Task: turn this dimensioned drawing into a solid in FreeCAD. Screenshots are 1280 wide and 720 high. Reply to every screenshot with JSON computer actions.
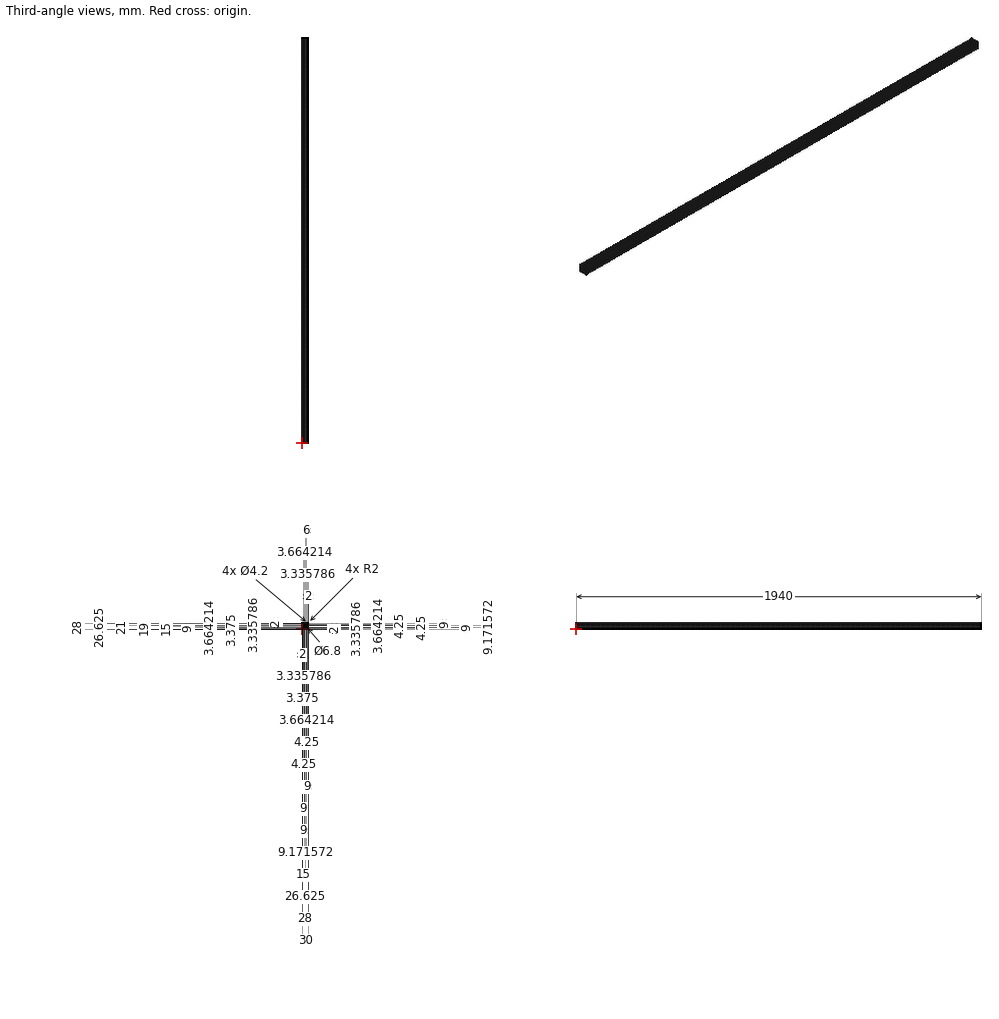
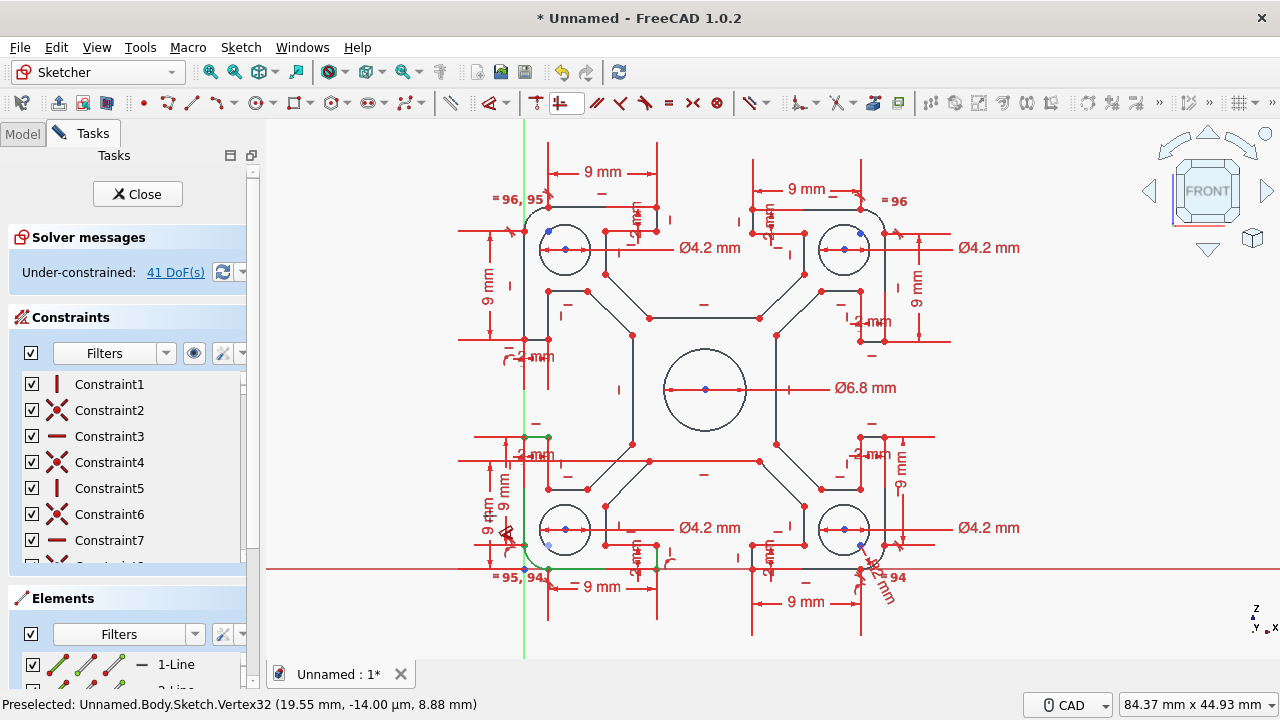
{"action": "left_click", "coordinate": [633, 445]}
{"action": "left_click", "coordinate": [579, 411]}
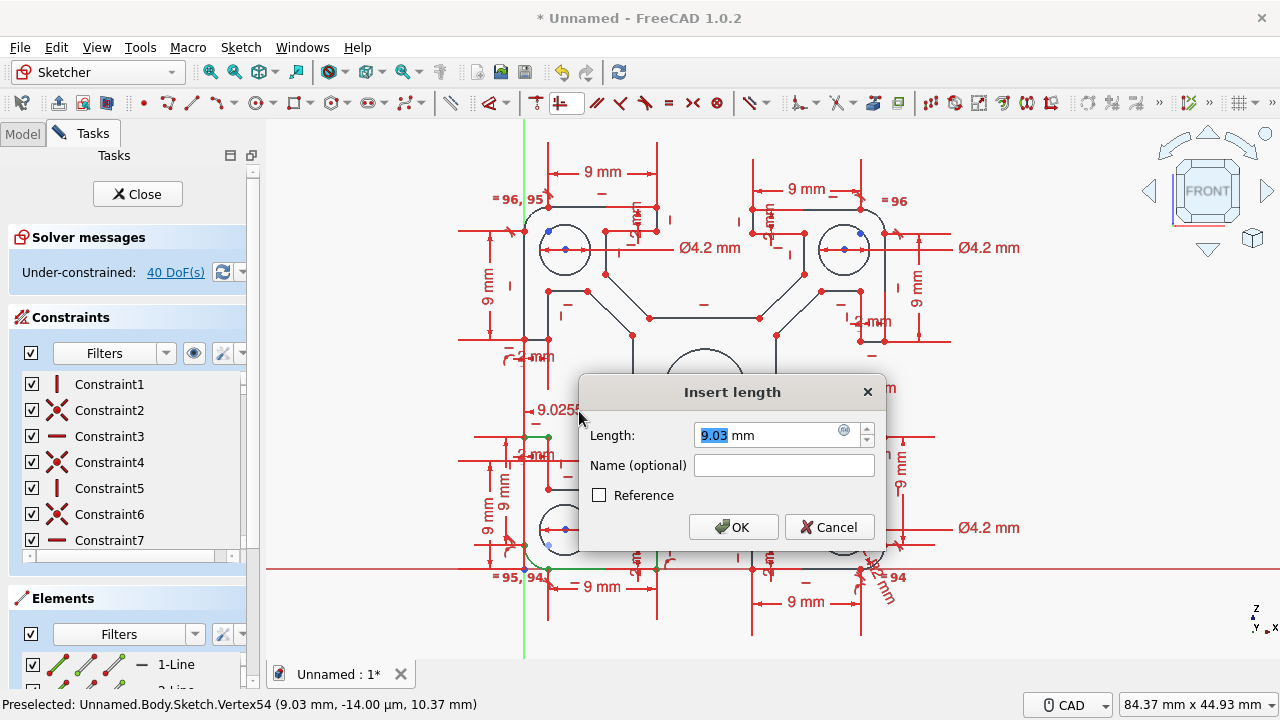
{"action": "type", "text": "9"}
{"action": "key", "text": "Return"}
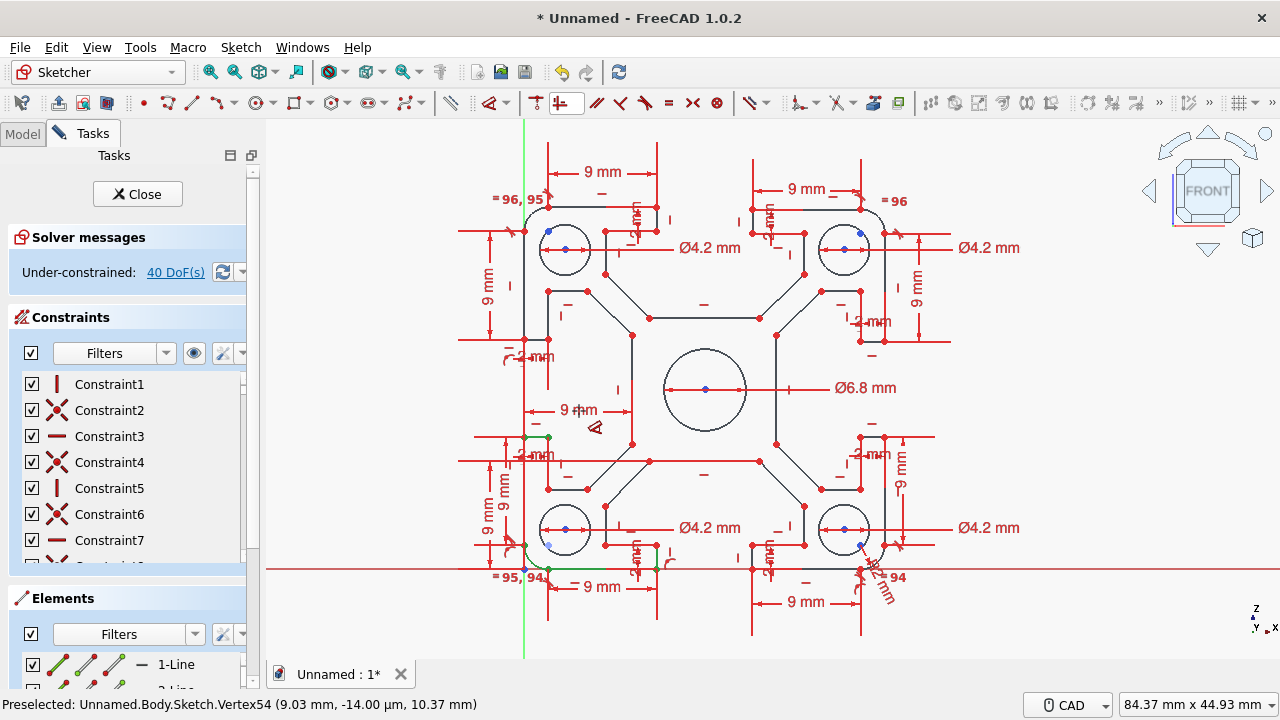
{"action": "left_click", "coordinate": [705, 390]}
{"action": "left_click", "coordinate": [678, 603]}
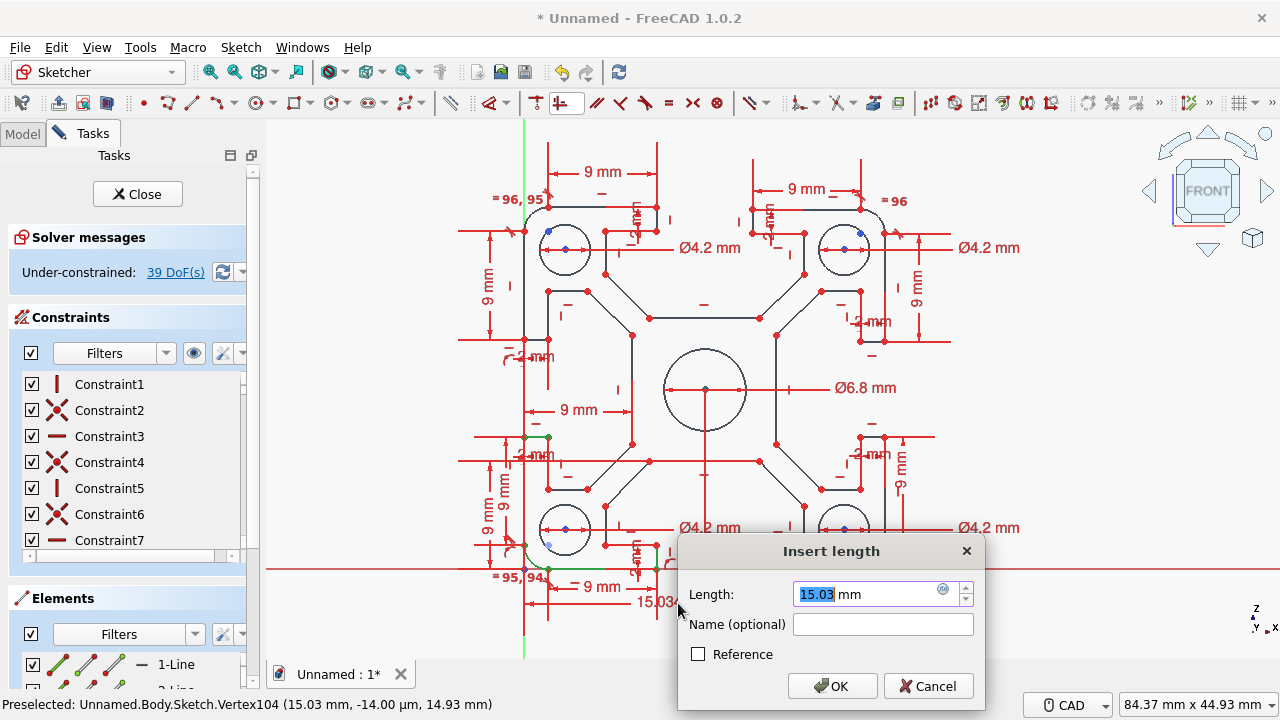
{"action": "type", "text": "15"}
{"action": "key", "text": "Return"}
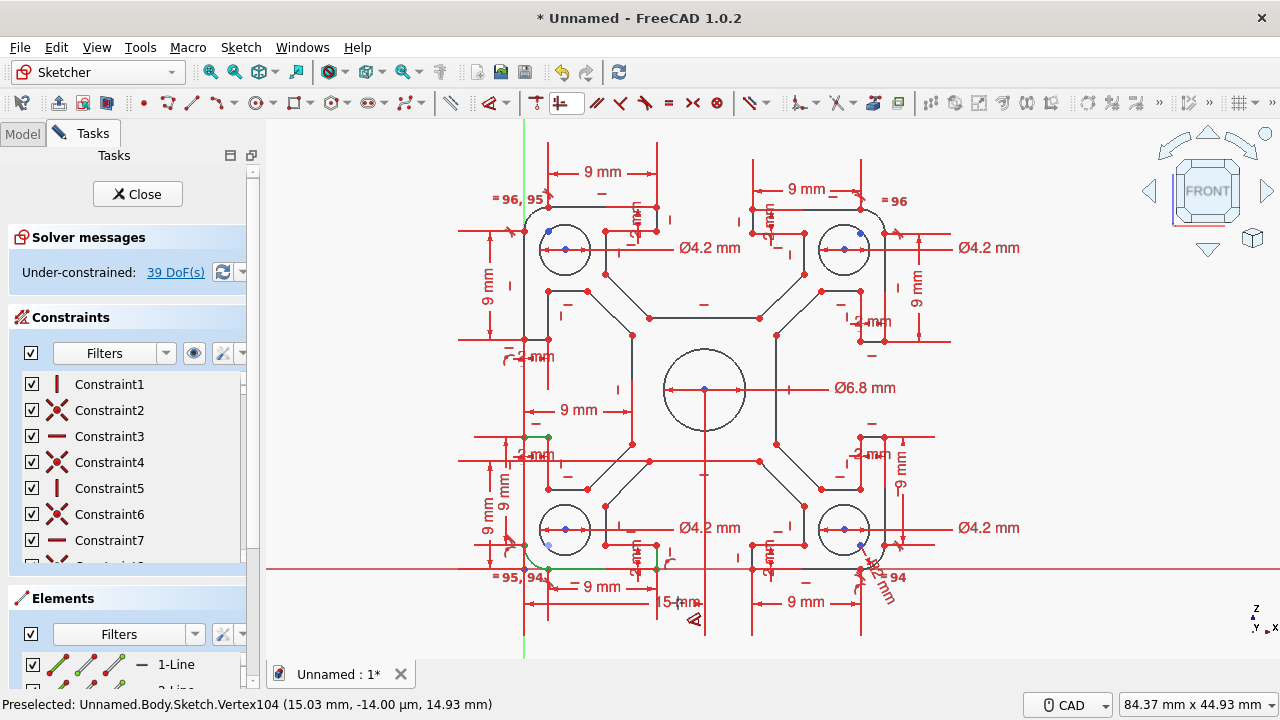
{"action": "left_click", "coordinate": [705, 390]}
{"action": "left_click", "coordinate": [490, 417]}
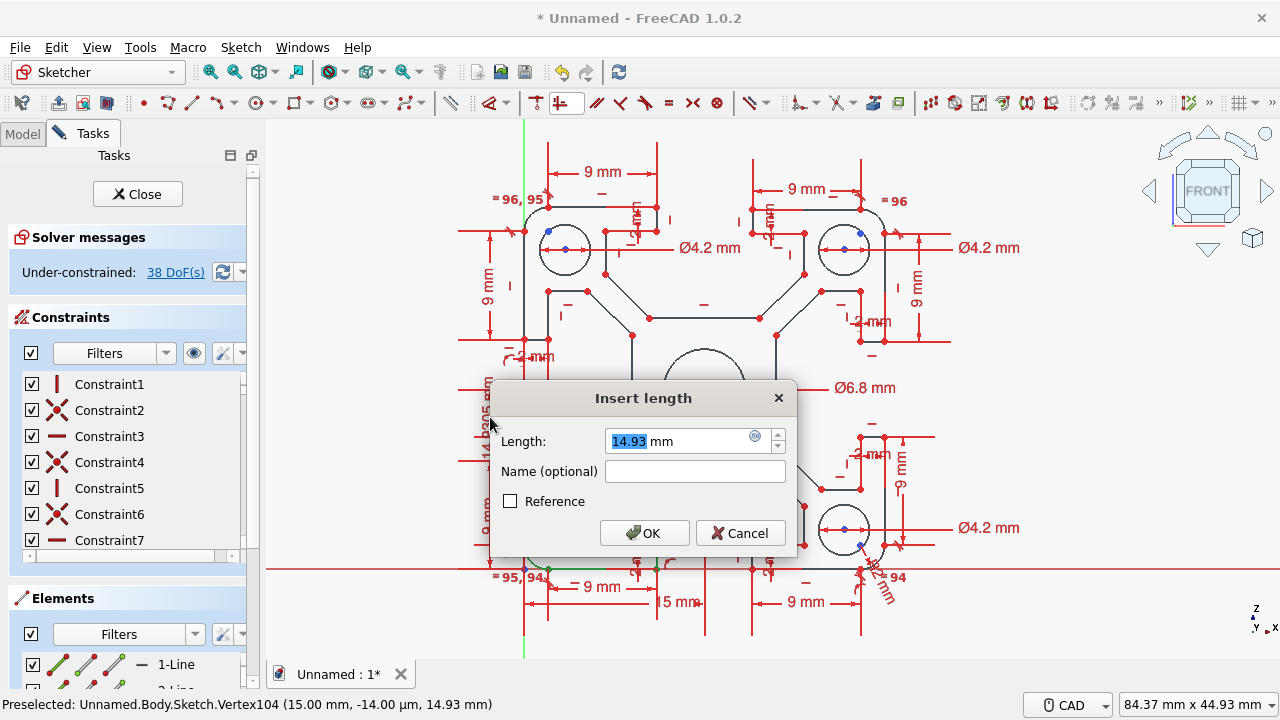
{"action": "type", "text": "15"}
{"action": "key", "text": "Return"}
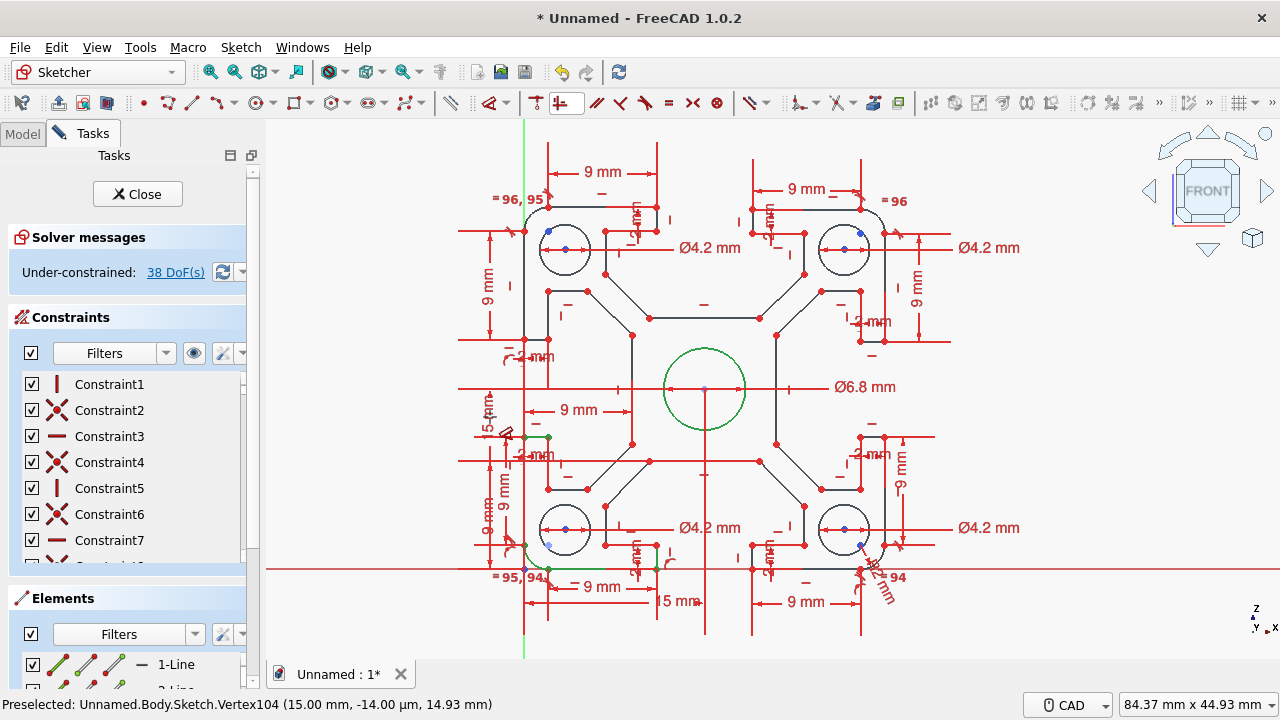
{"action": "left_click", "coordinate": [776, 335]}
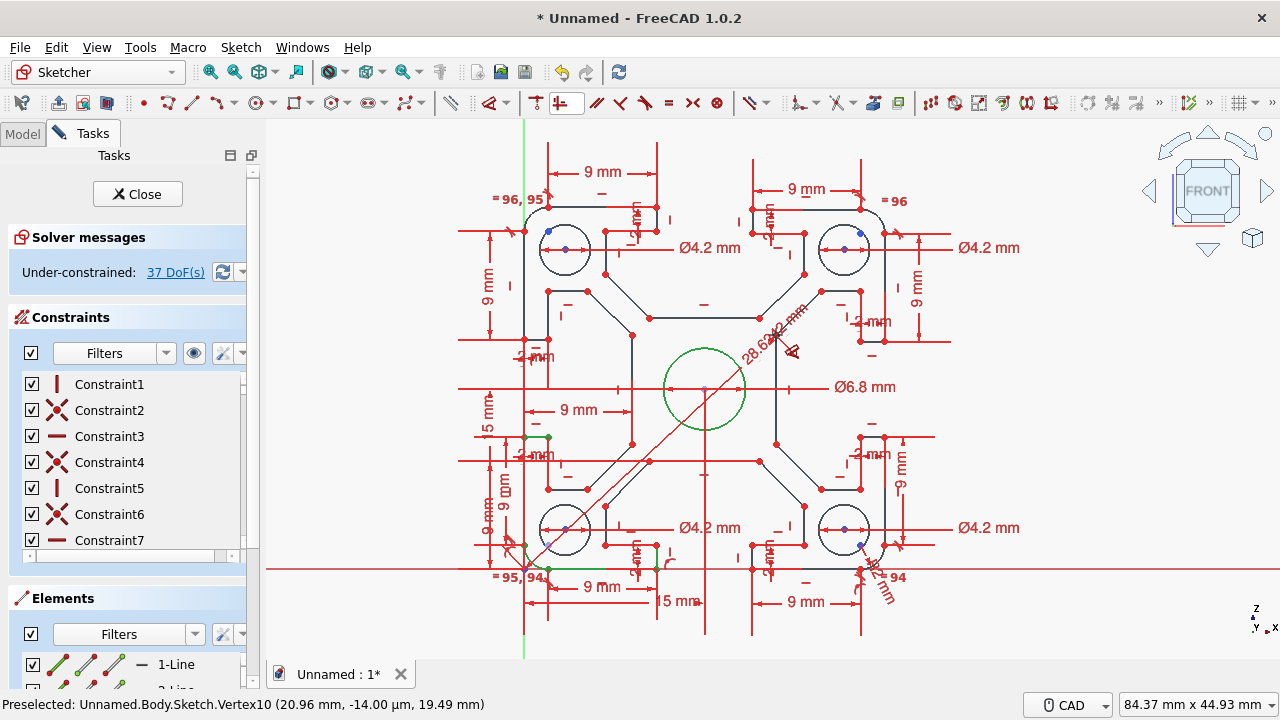
{"action": "left_click", "coordinate": [705, 389]}
{"action": "left_click", "coordinate": [740, 301]}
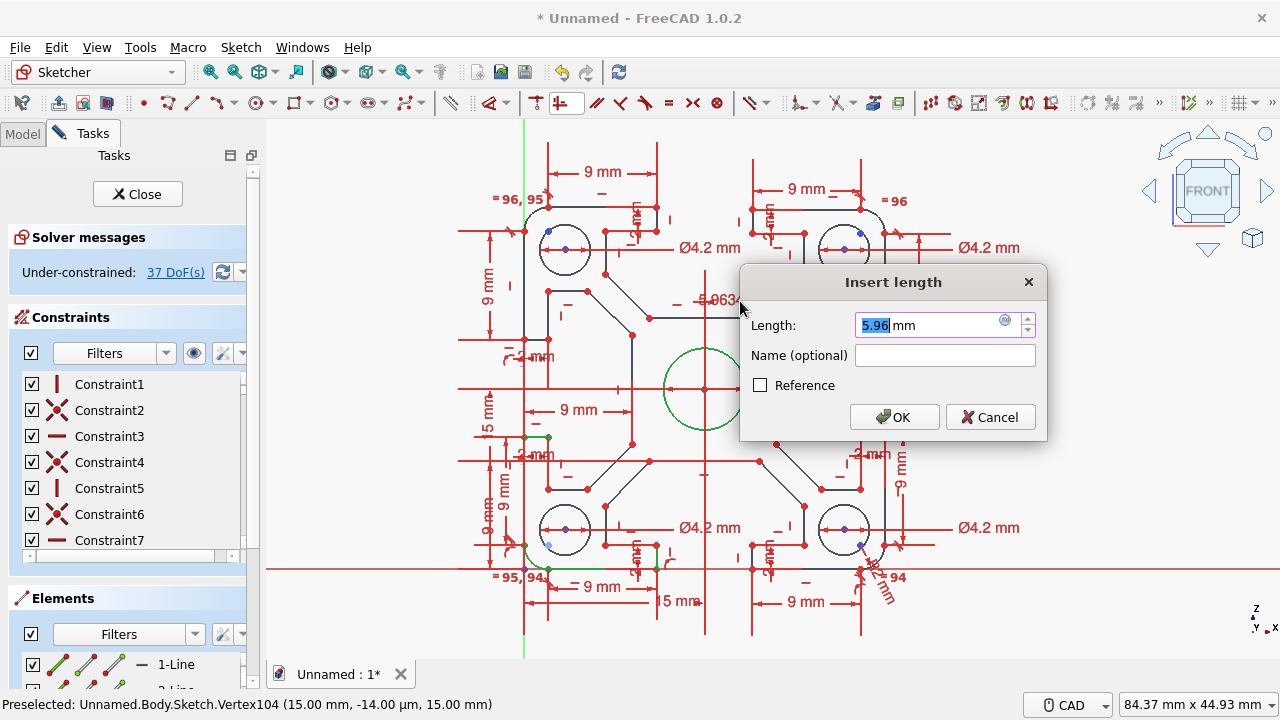
{"action": "type", "text": "6"}
{"action": "key", "text": "Return"}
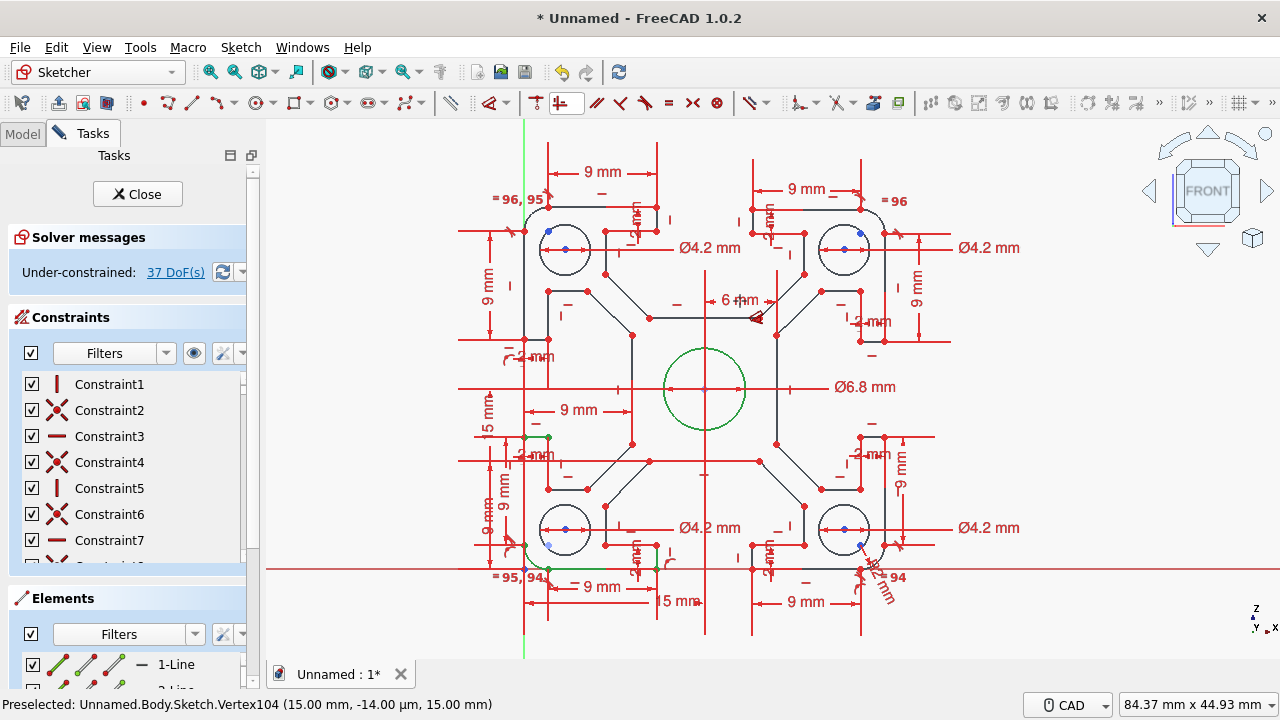
{"action": "left_click", "coordinate": [885, 234]}
{"action": "left_click", "coordinate": [705, 200]}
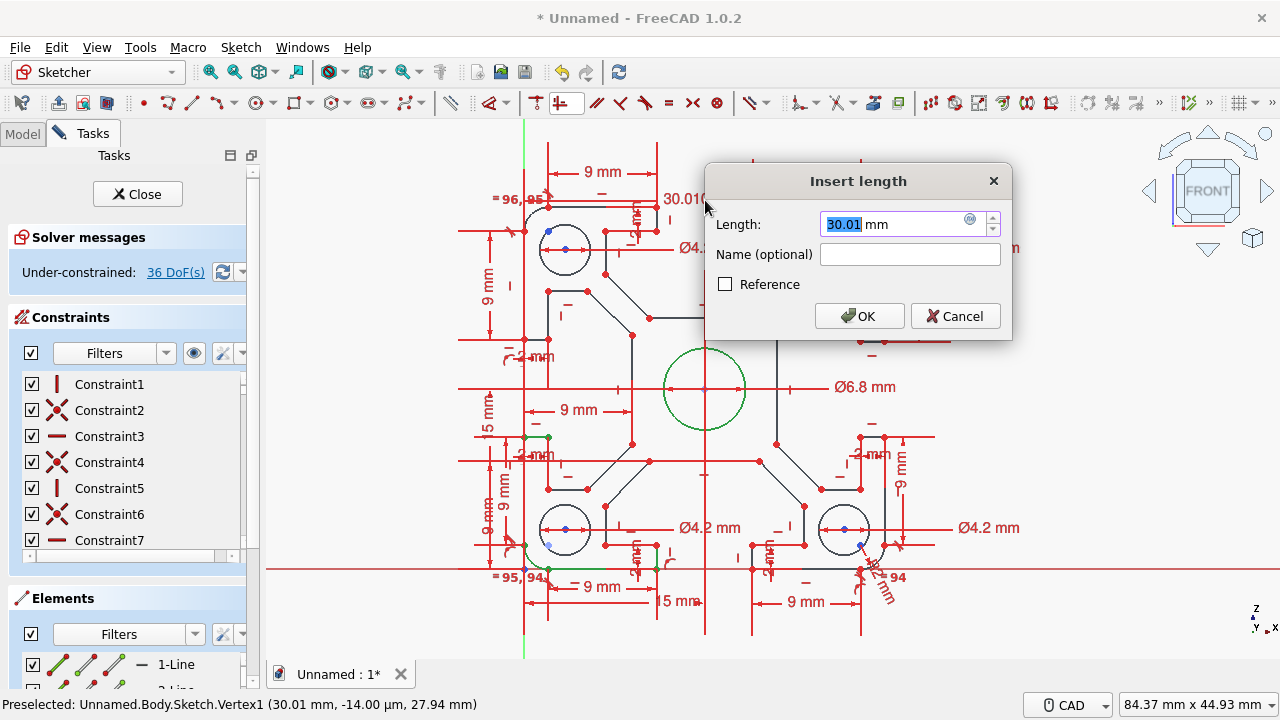
{"action": "type", "text": "30"}
{"action": "key", "text": "Return"}